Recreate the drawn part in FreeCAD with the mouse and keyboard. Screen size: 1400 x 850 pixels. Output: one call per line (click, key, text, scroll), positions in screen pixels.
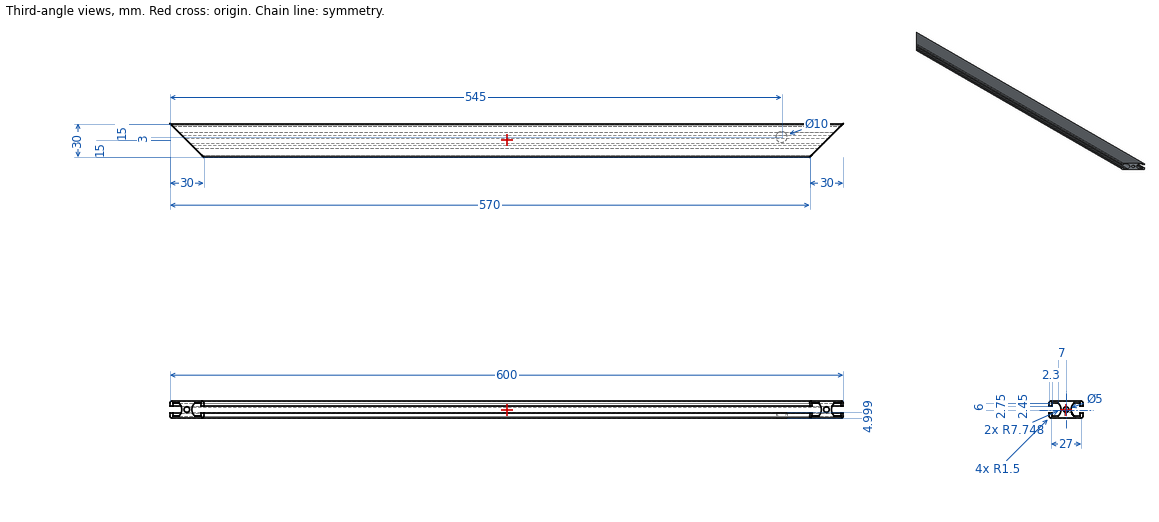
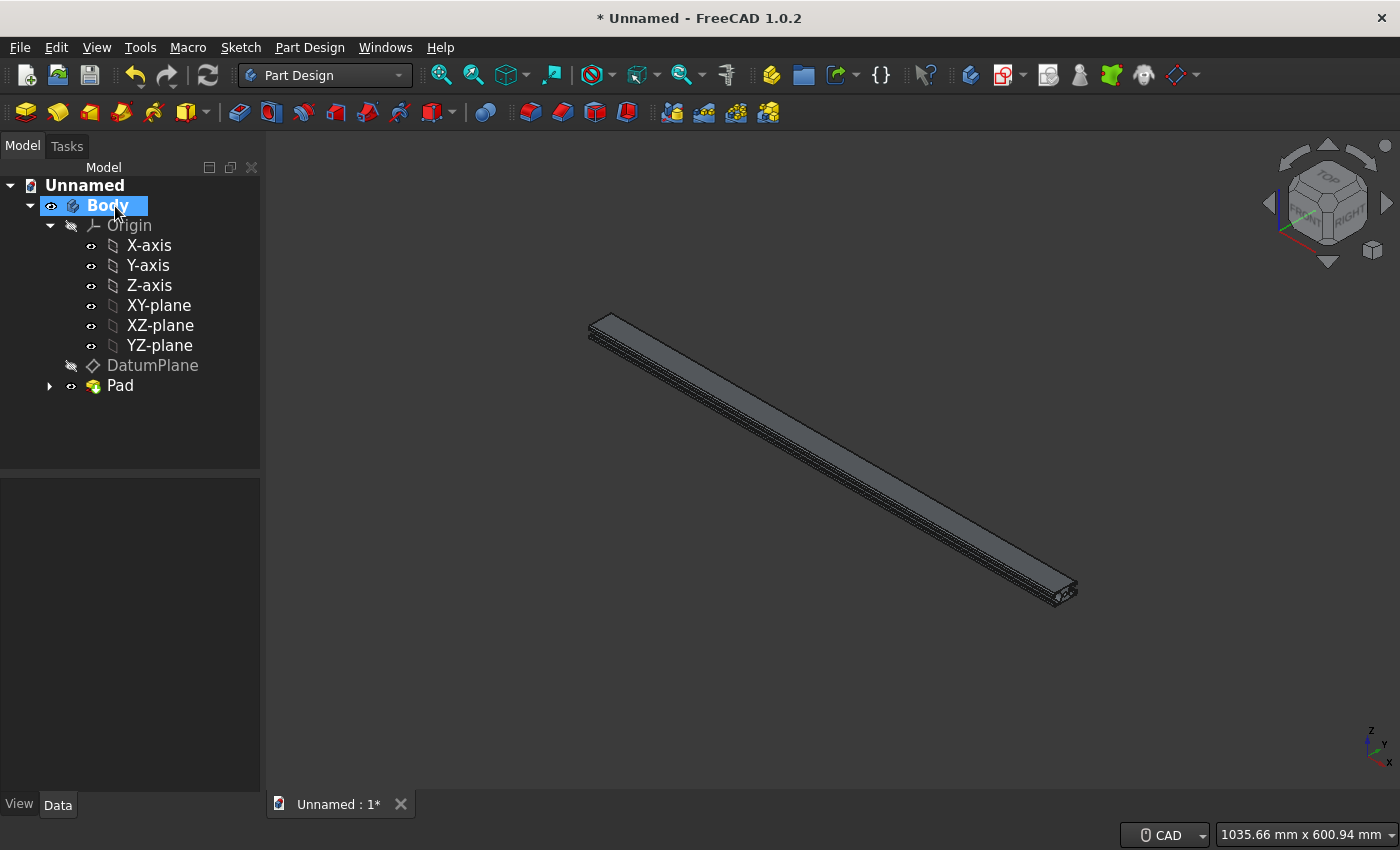
click(442, 76)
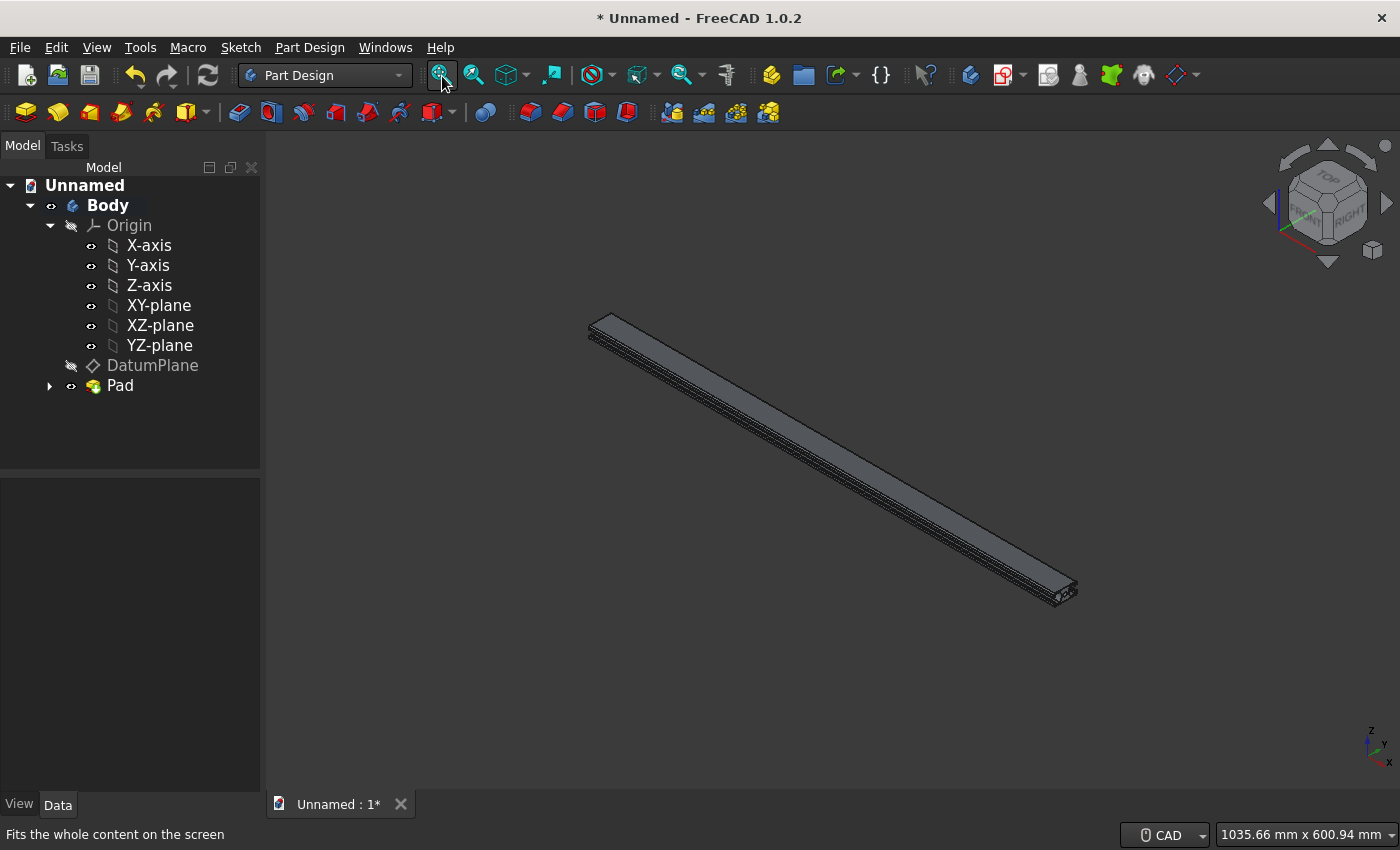
click(899, 491)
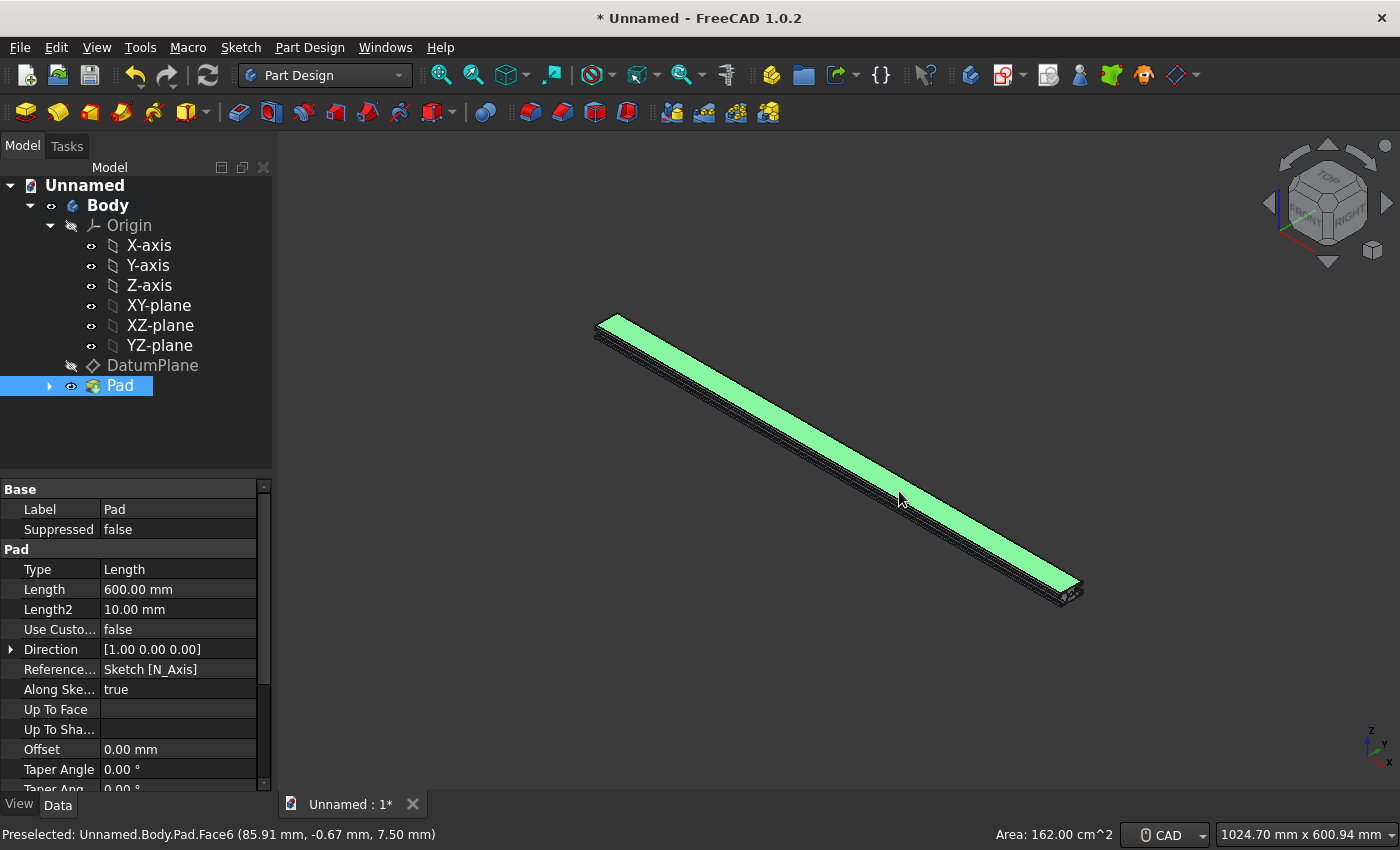
click(1004, 76)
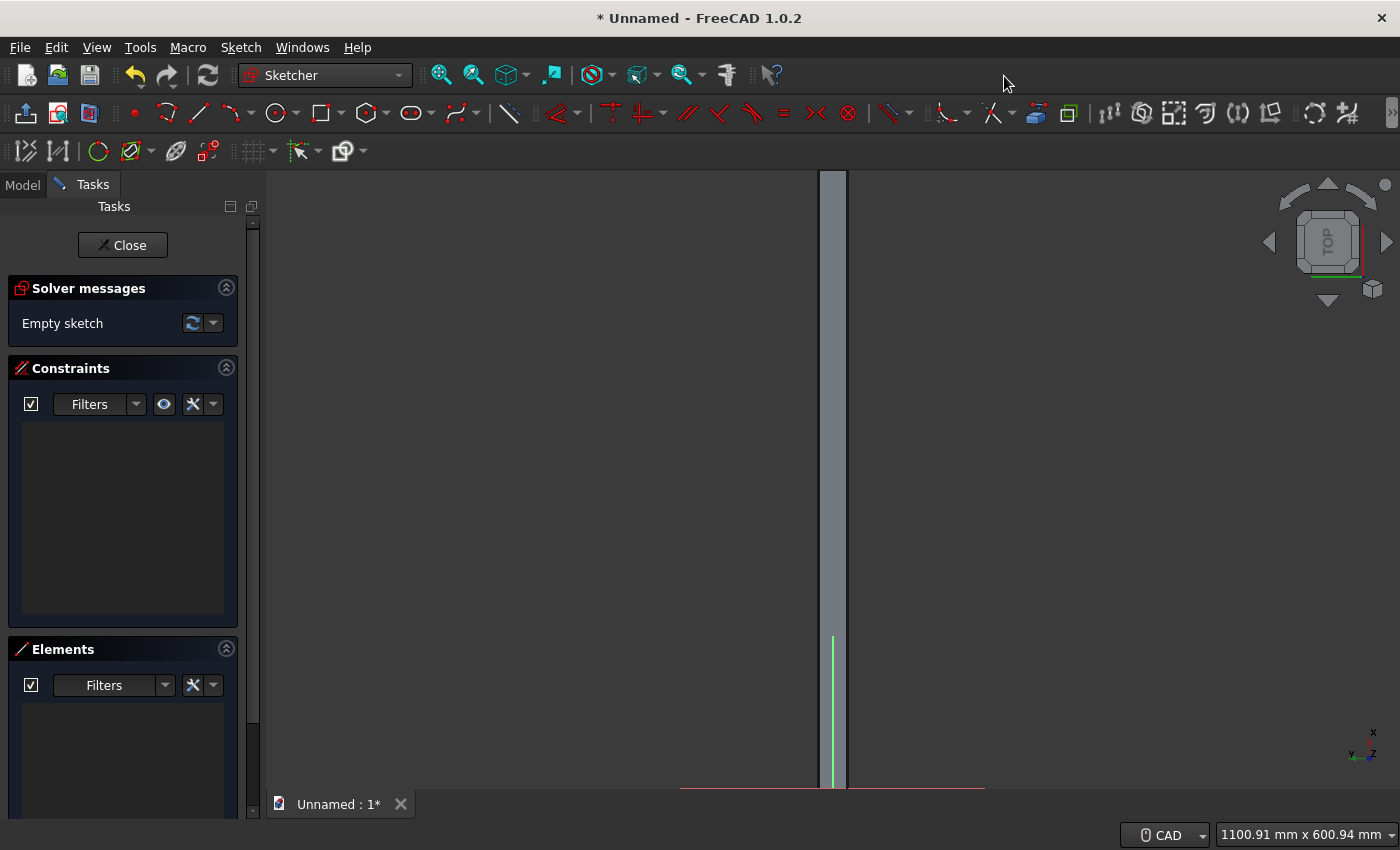
scroll(625, 480, down, 2)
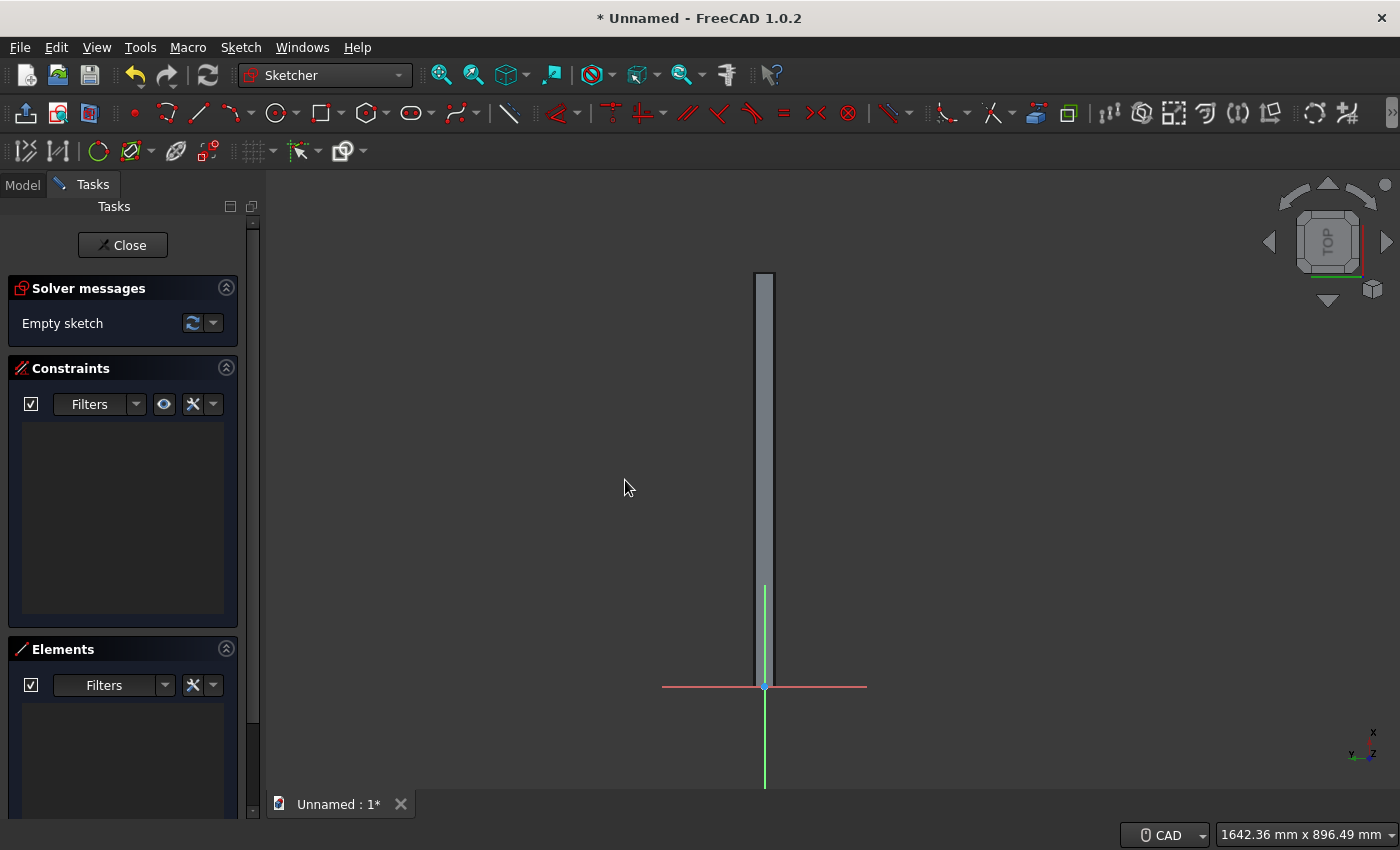
key(g)
key(m)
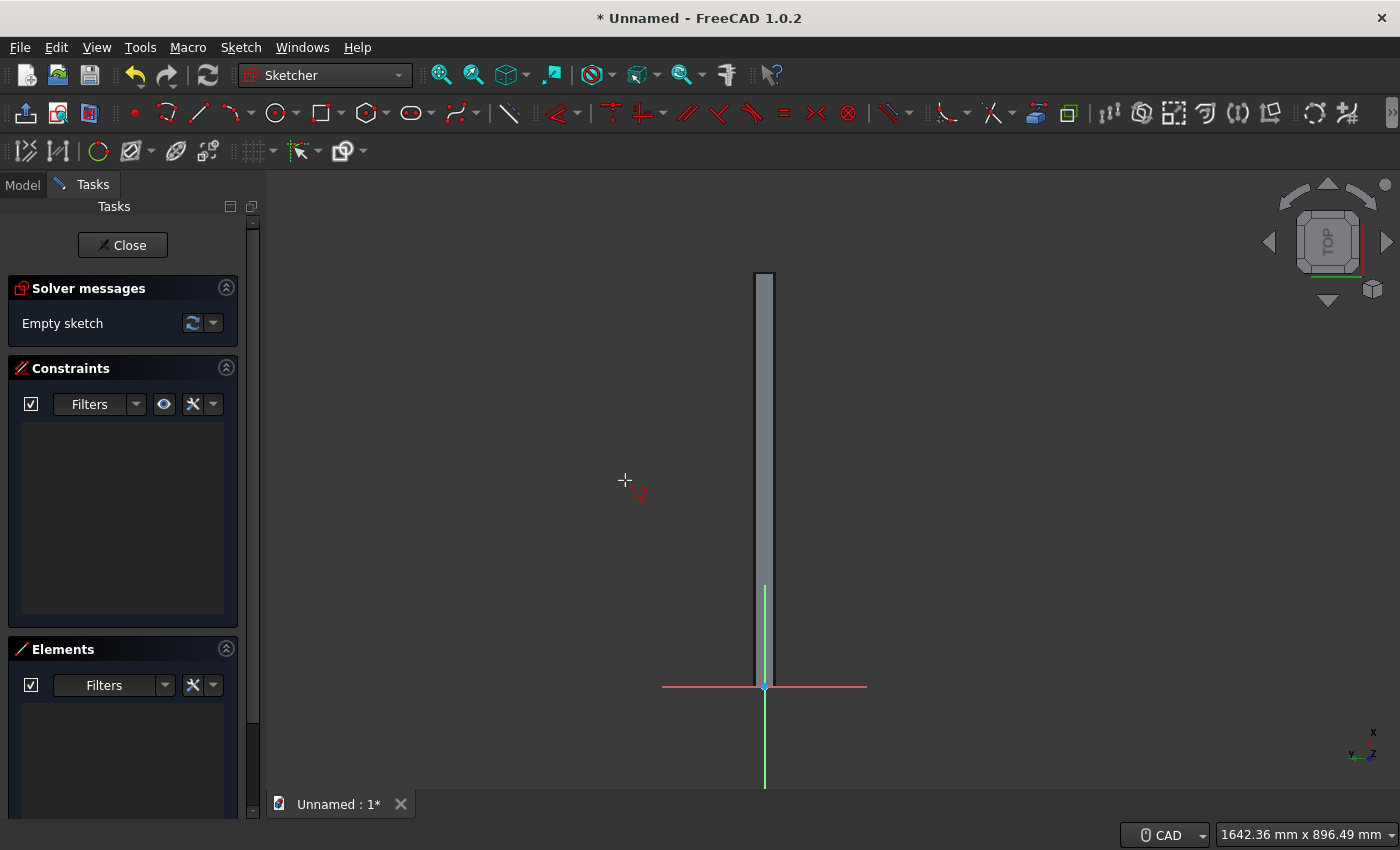
scroll(754, 687, up, 3)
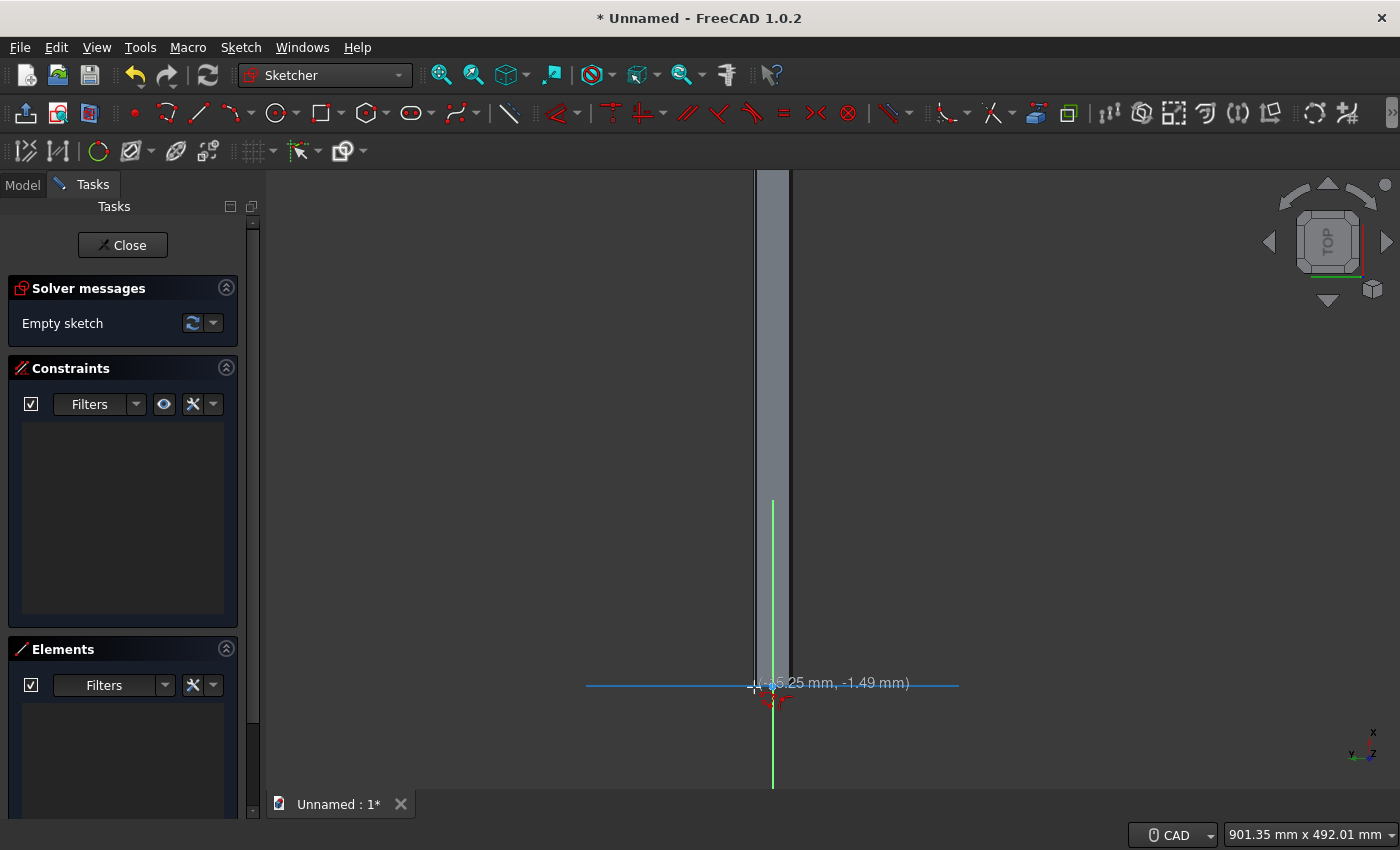
click(754, 686)
click(792, 677)
click(792, 649)
click(754, 686)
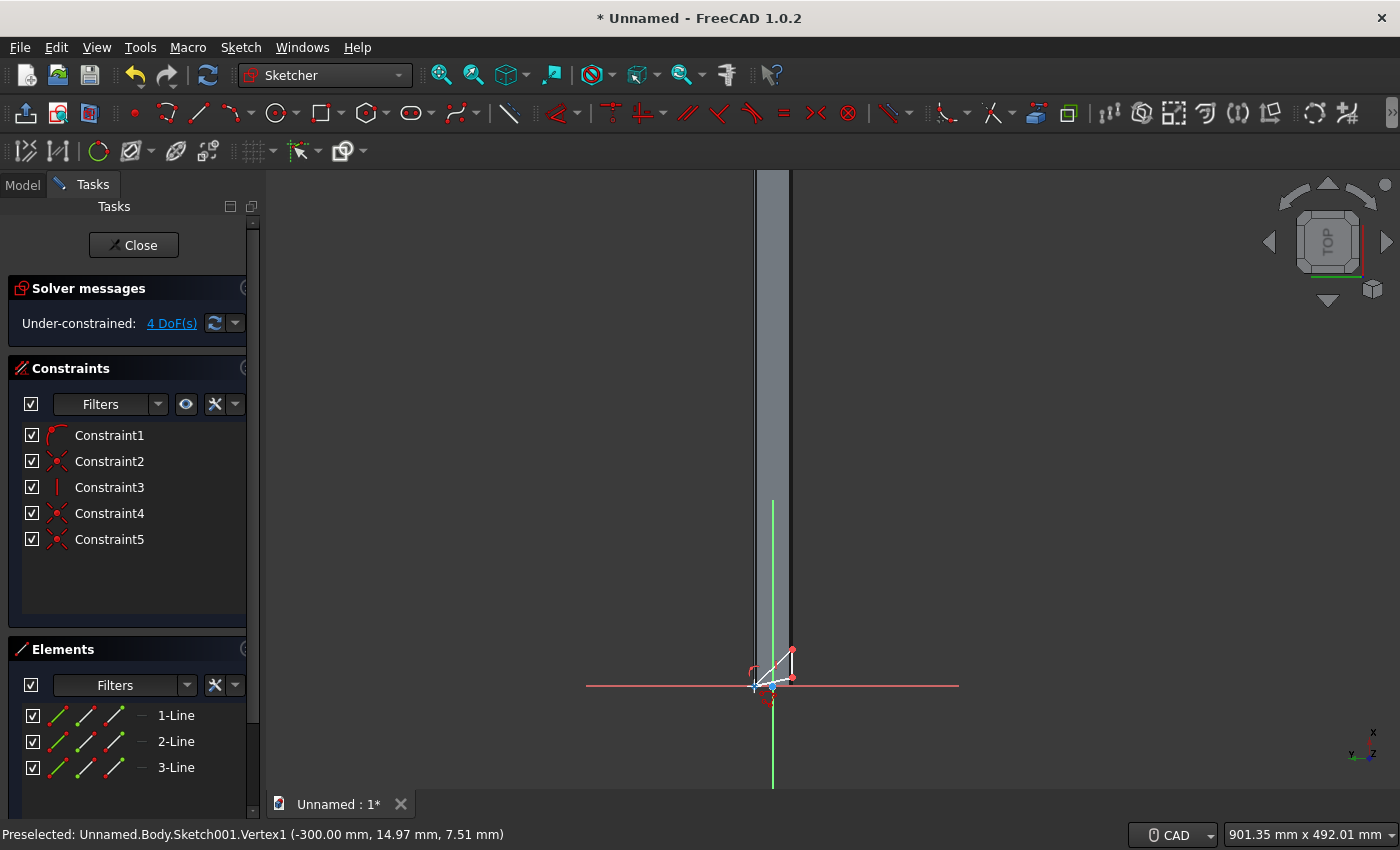
scroll(754, 687, down, 3)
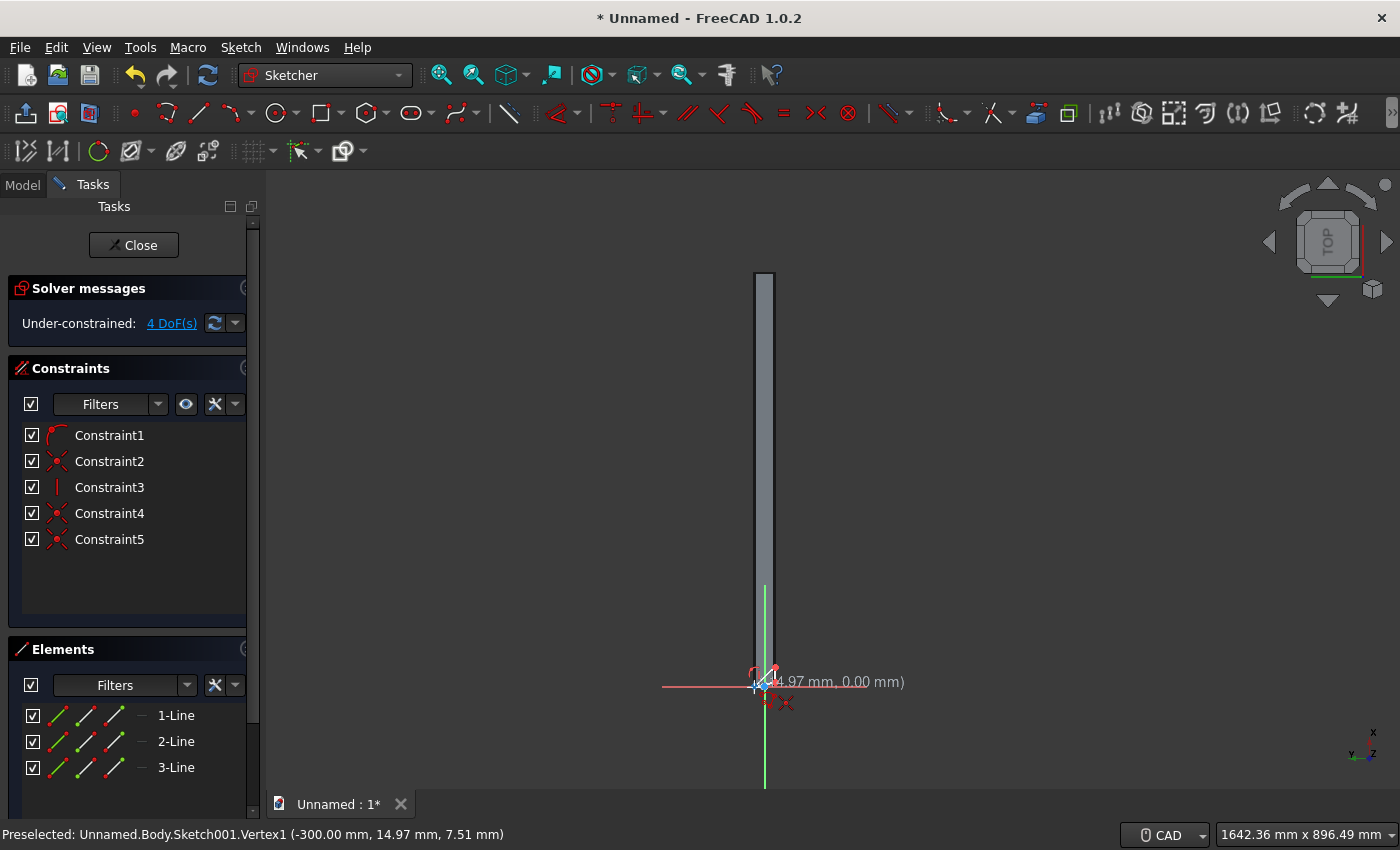
scroll(775, 293, up, 3)